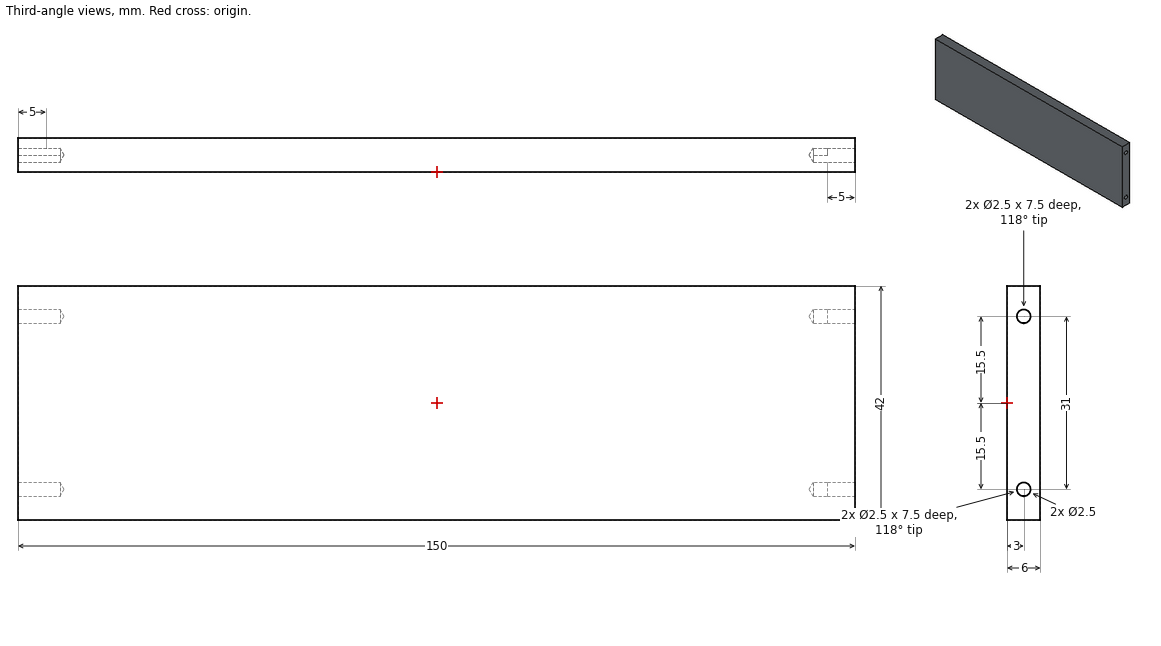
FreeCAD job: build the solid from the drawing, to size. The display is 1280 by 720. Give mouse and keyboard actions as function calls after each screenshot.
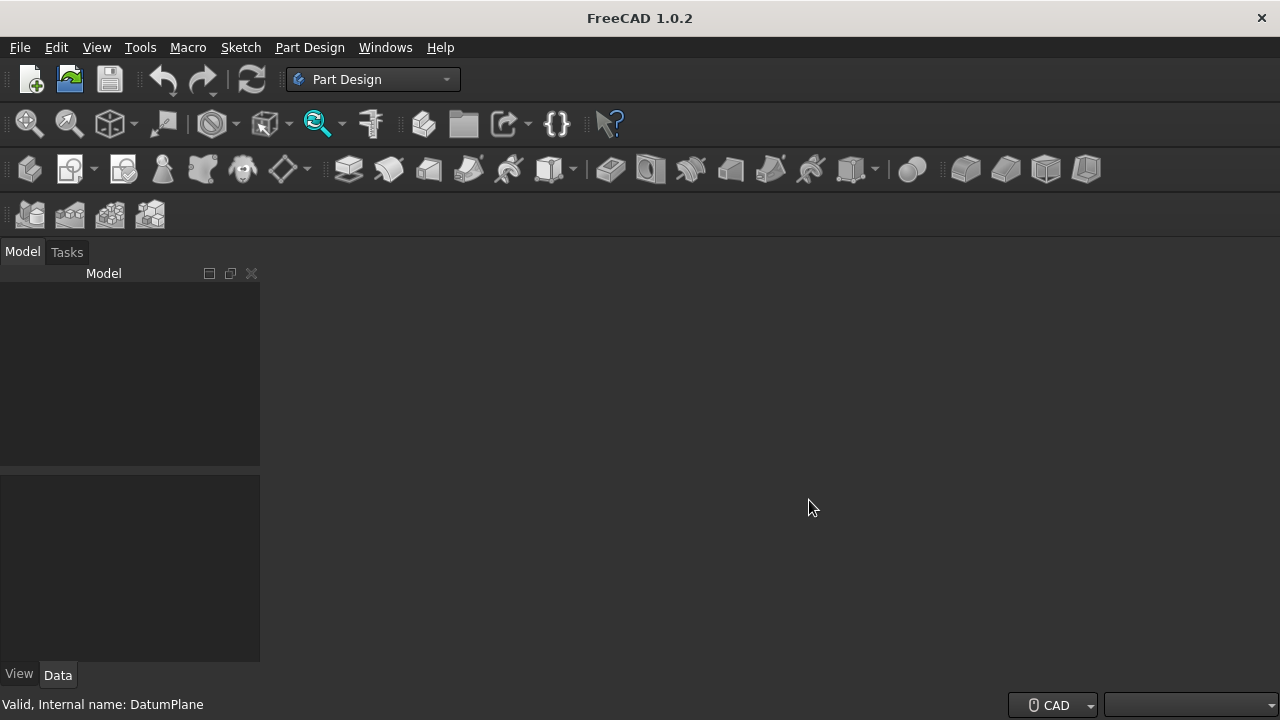
click(30, 80)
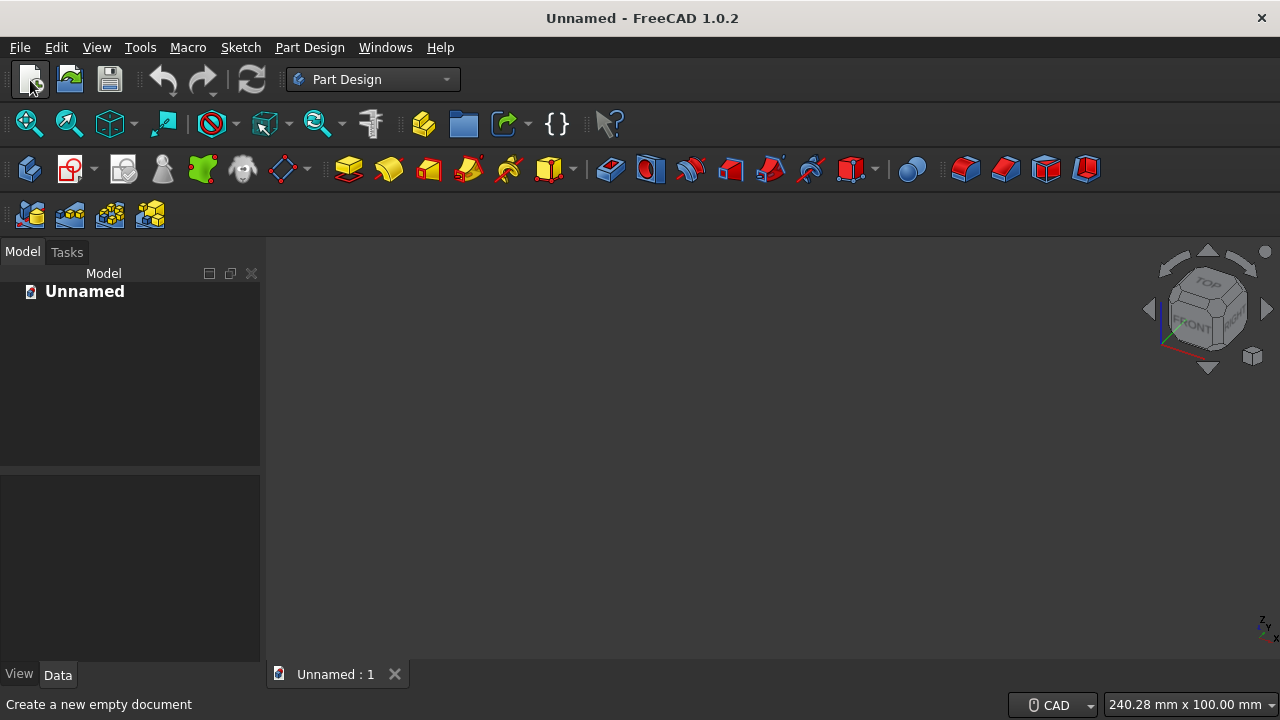
click(70, 170)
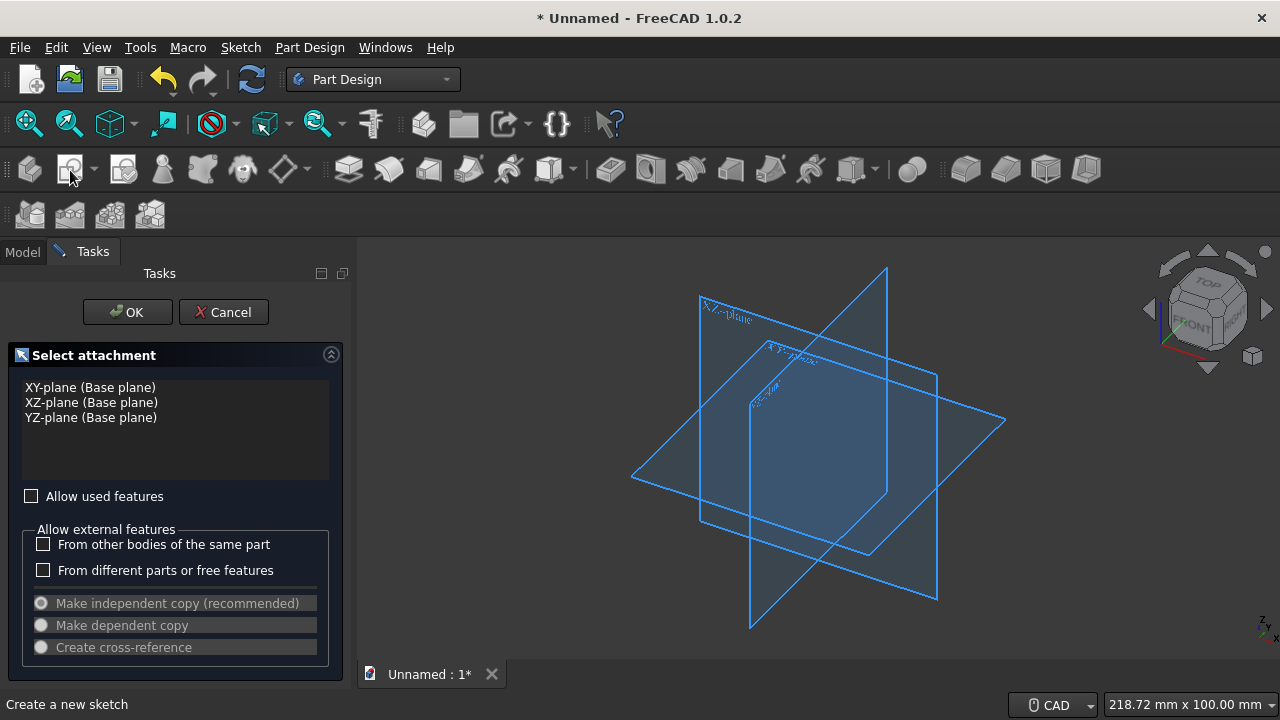
click(82, 402)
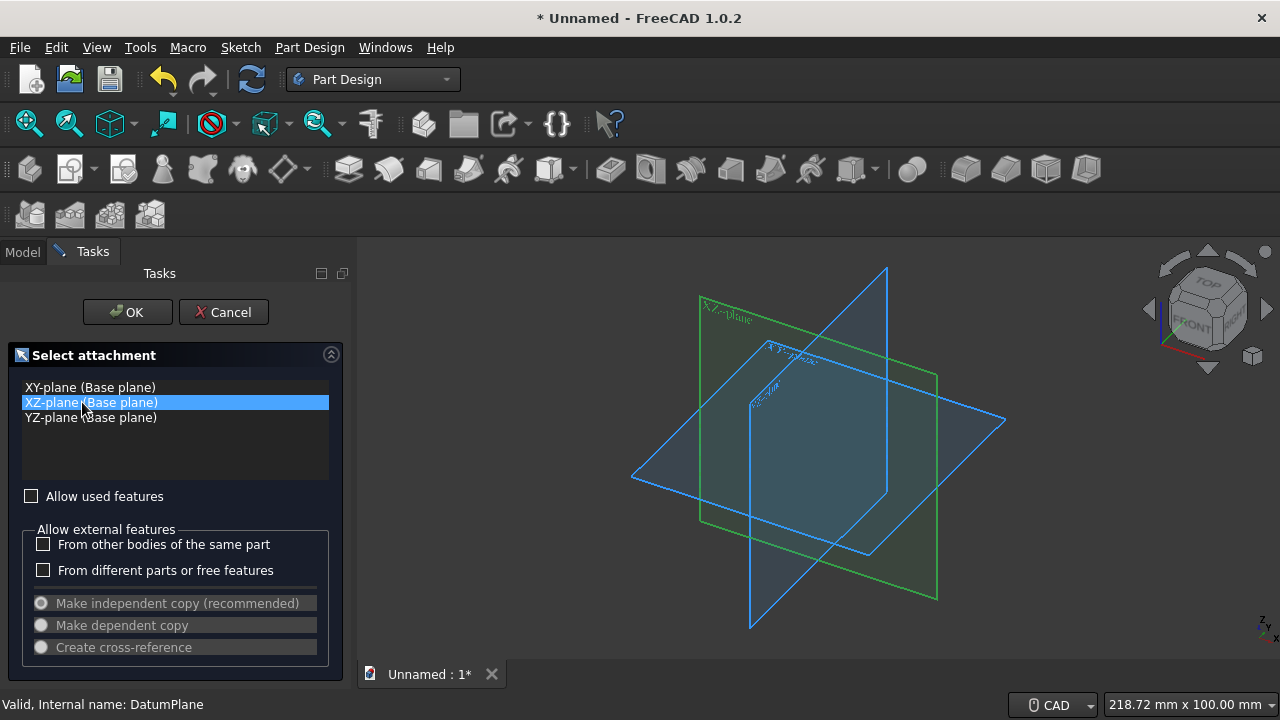
click(128, 312)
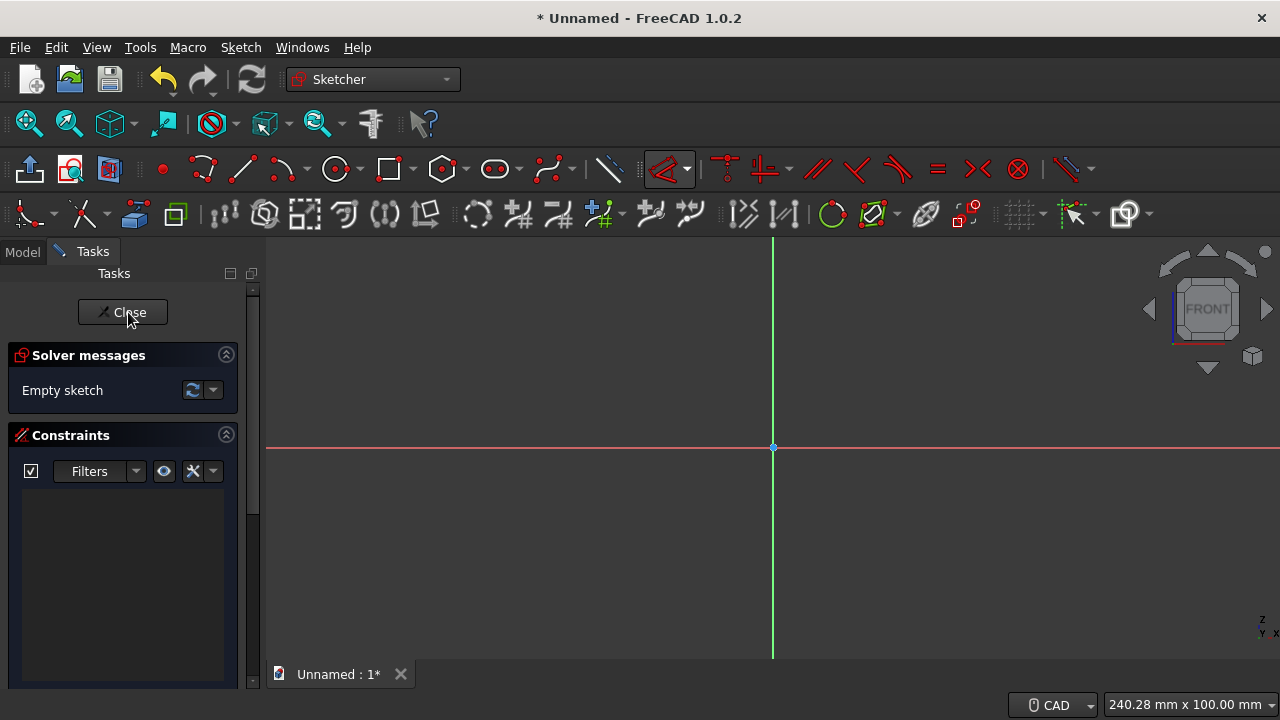
key(g)
key(v)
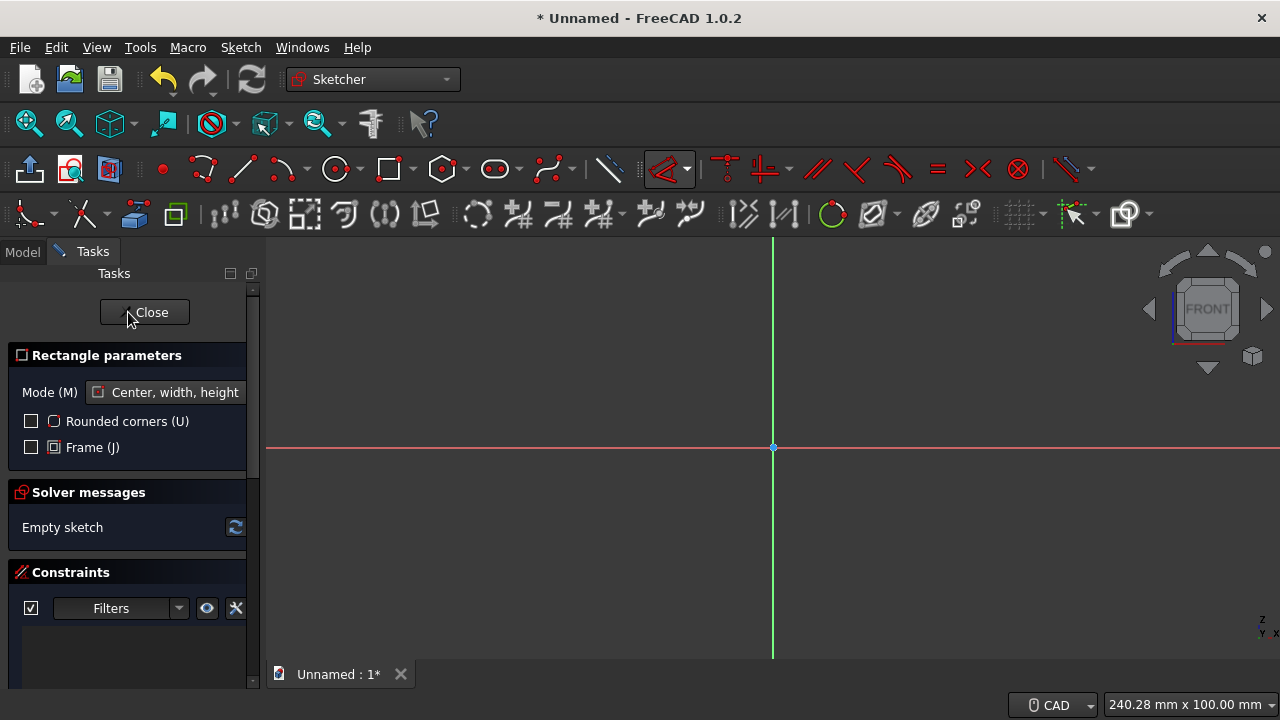
click(773, 448)
move(1090, 359)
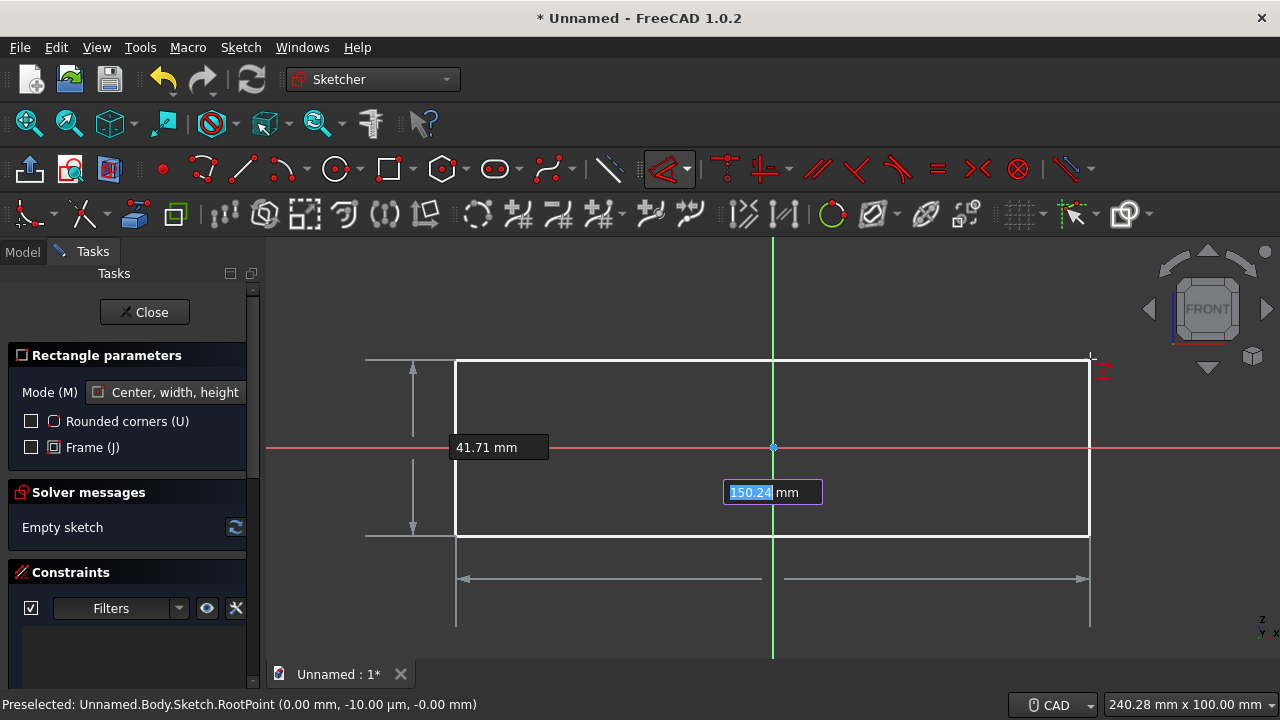
text(150)
key(Tab)
text(42)
key(Return)
key(Escape)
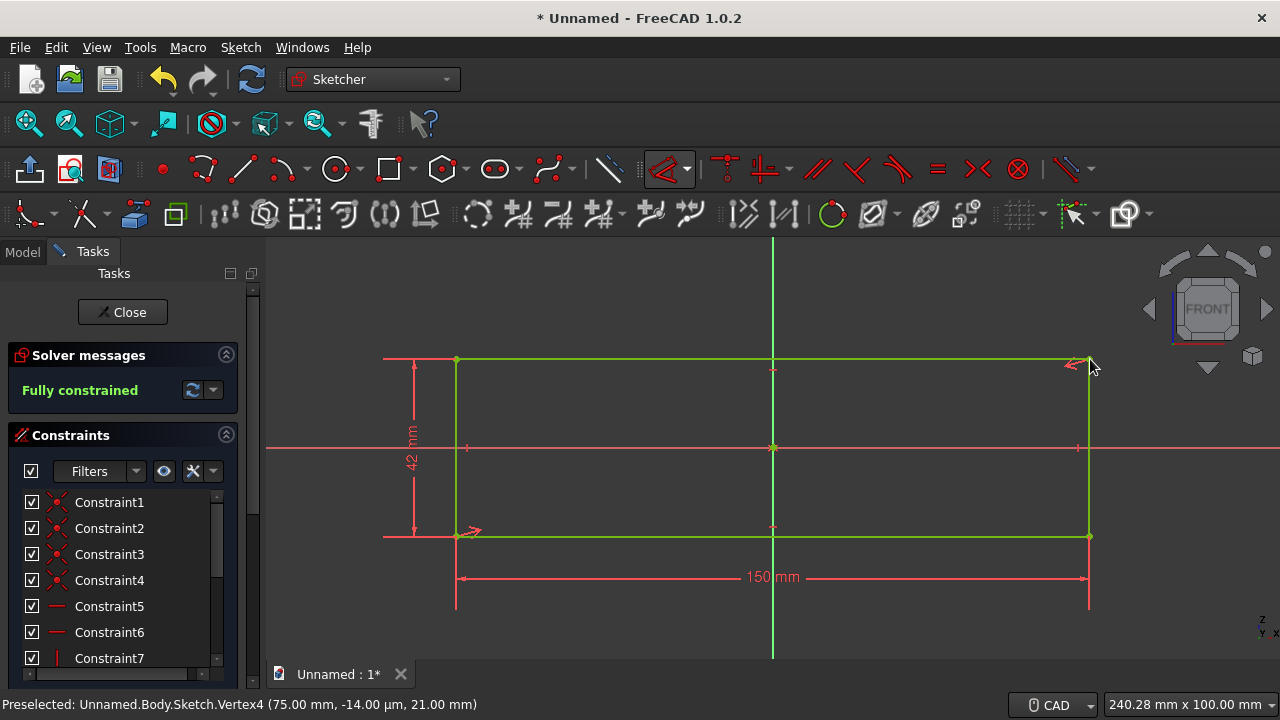
click(123, 312)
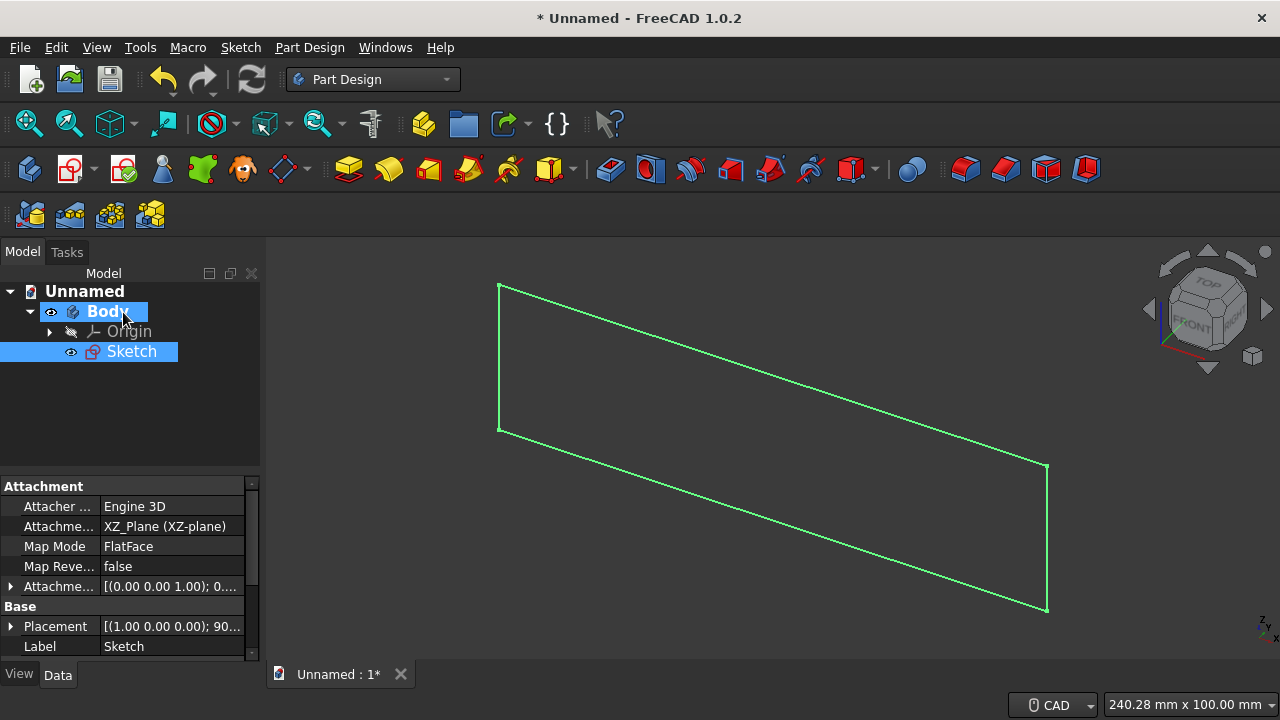
click(350, 170)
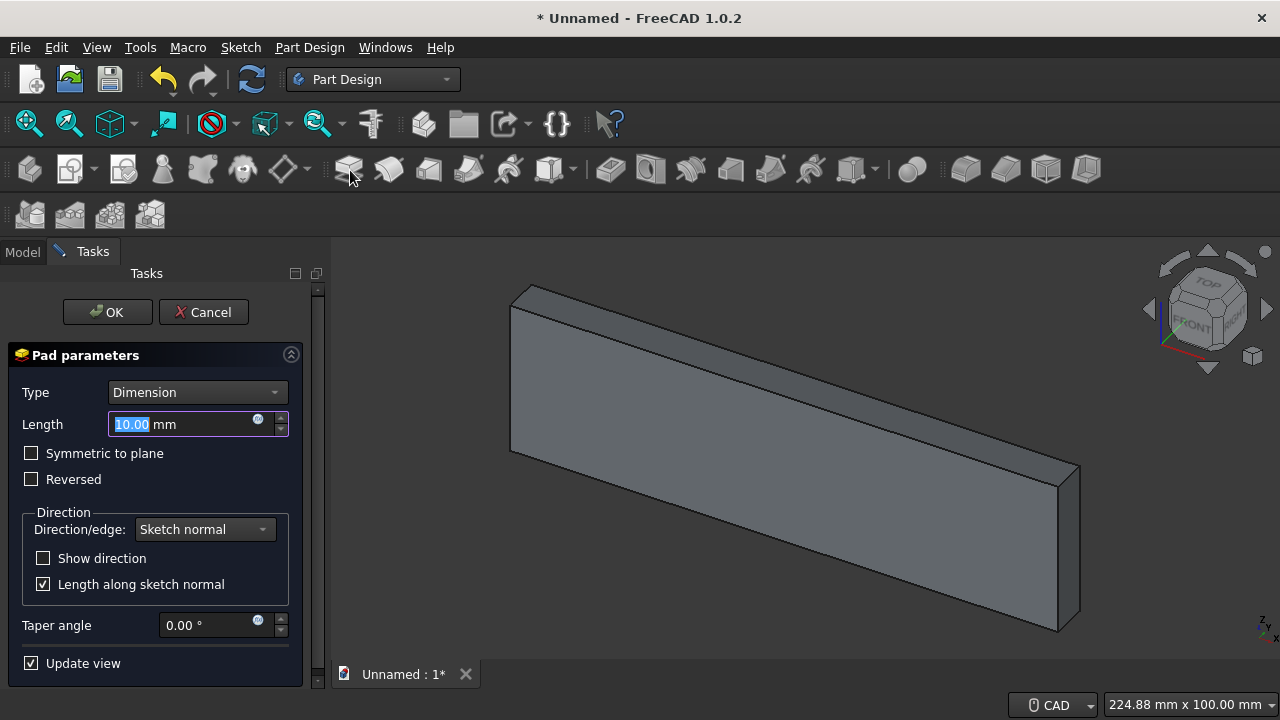
text(6)
key(Tab)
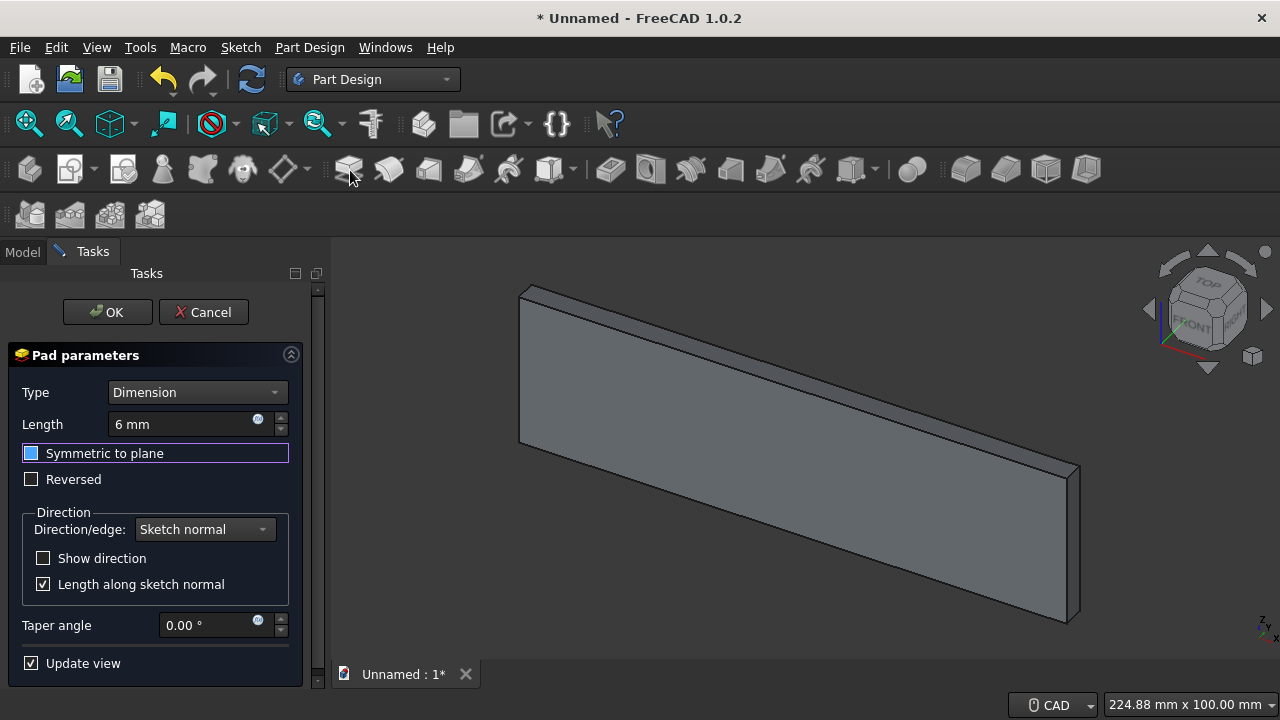
click(30, 479)